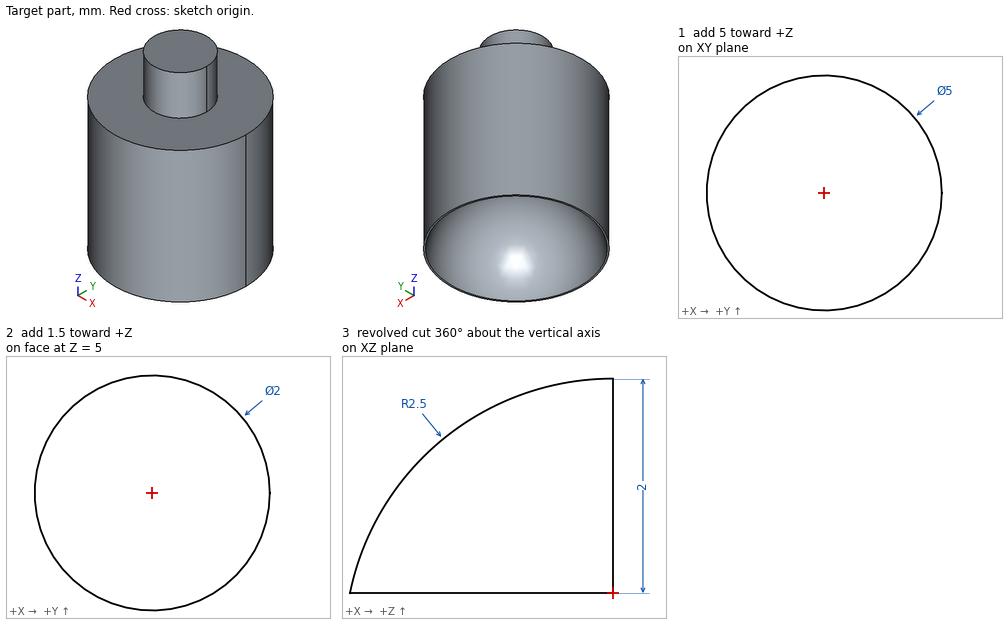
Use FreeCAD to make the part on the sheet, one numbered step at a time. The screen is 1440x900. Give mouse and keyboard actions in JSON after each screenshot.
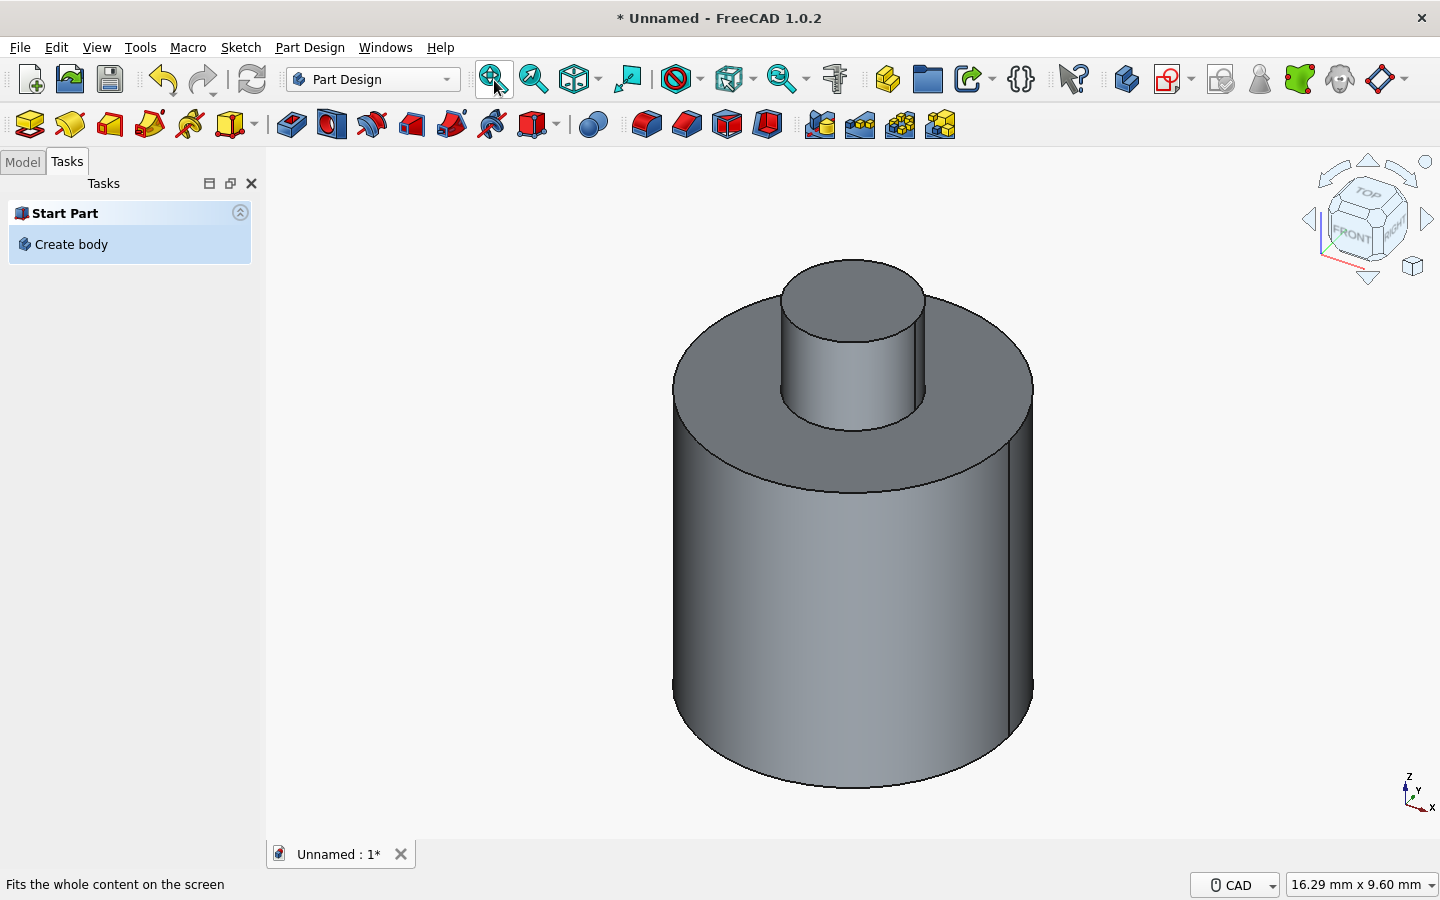
{"action": "left_click", "coordinate": [1168, 80]}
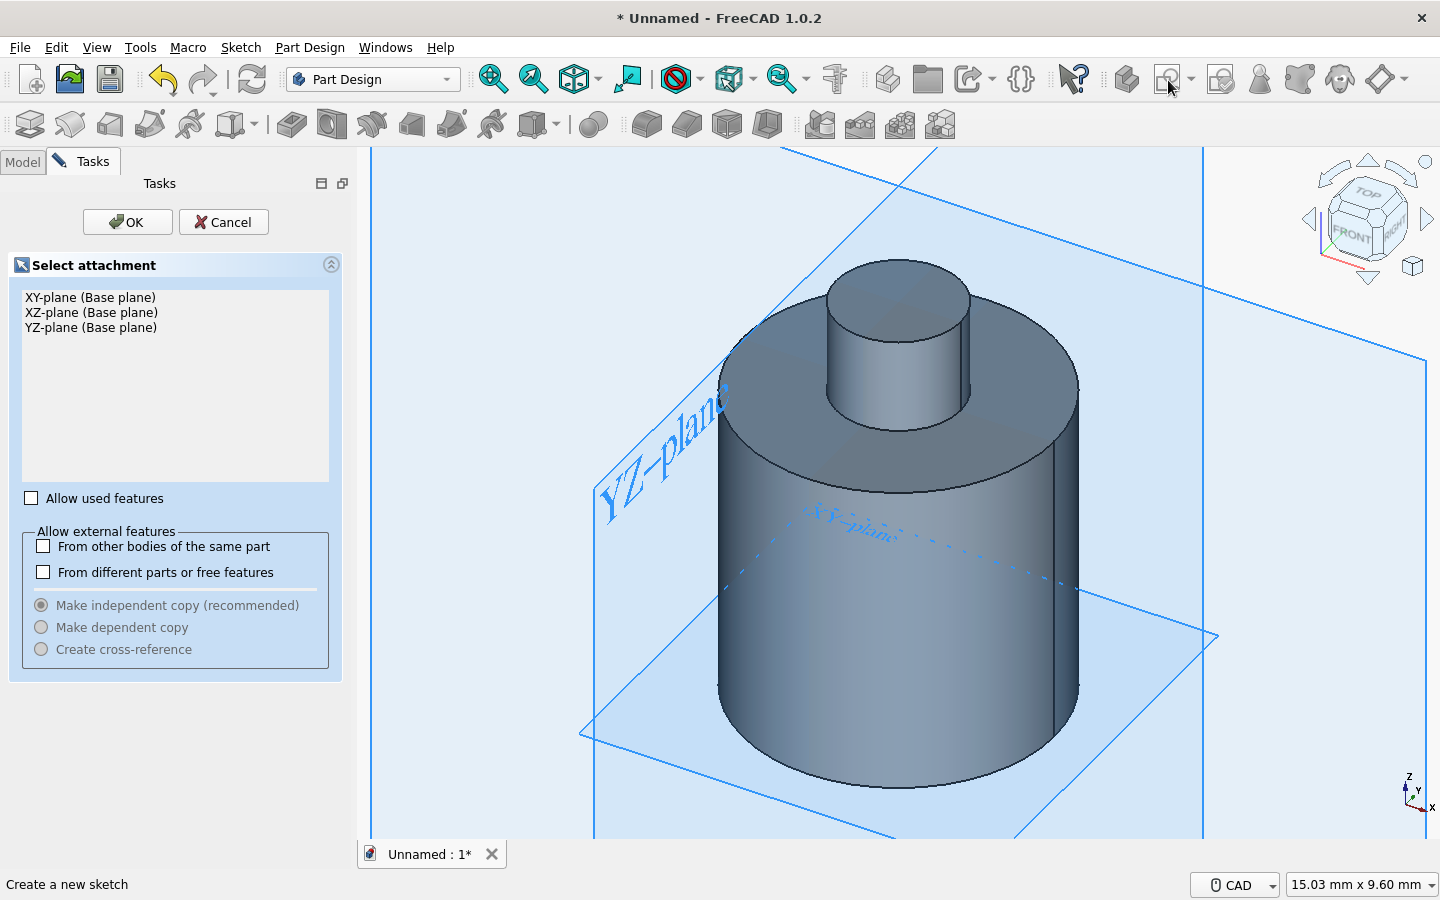
{"action": "left_click", "coordinate": [82, 312]}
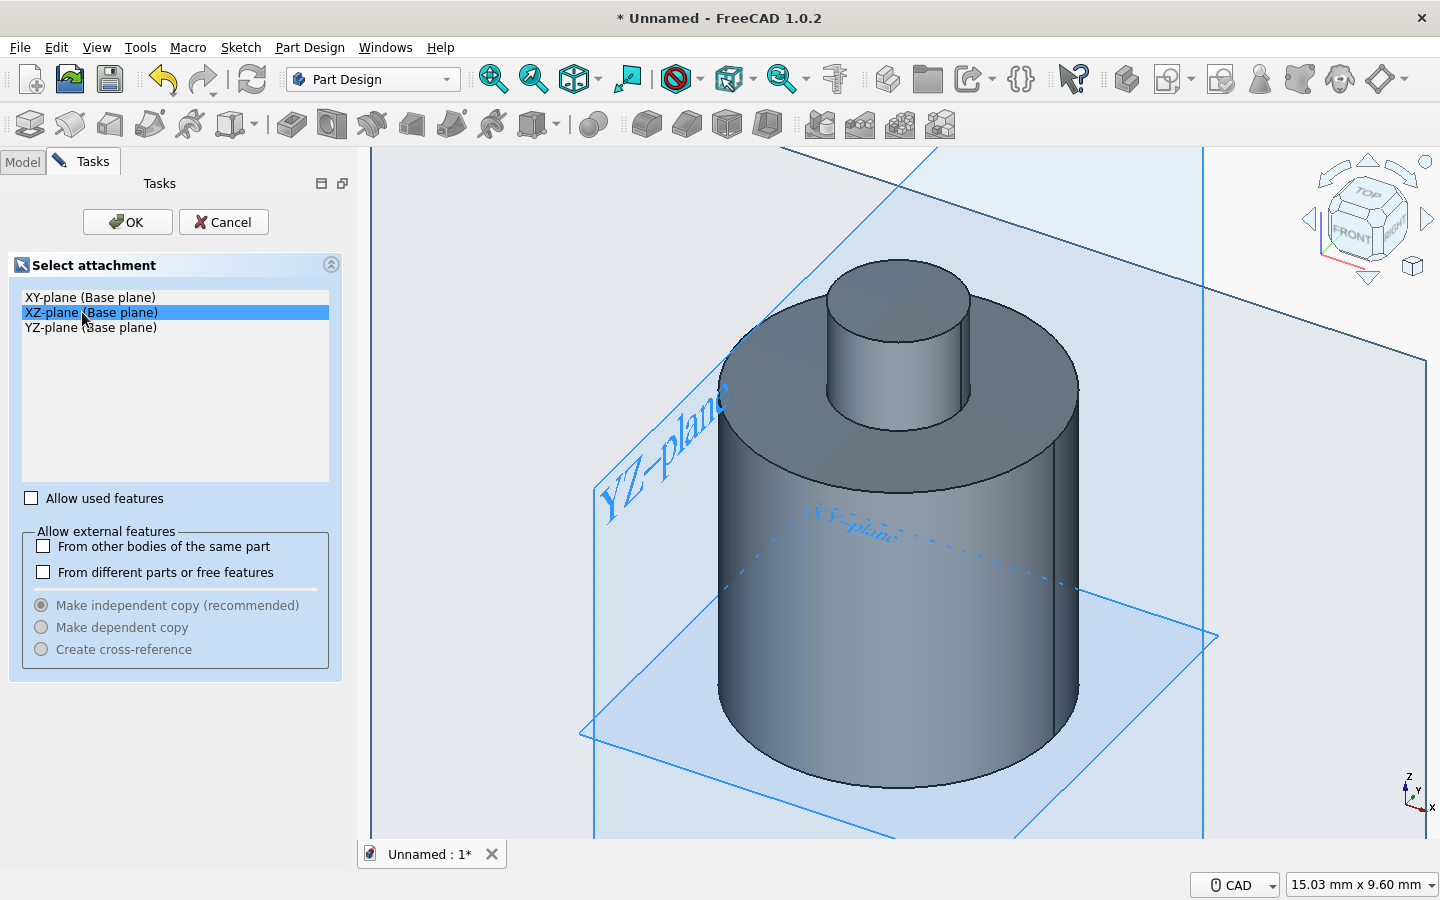
{"action": "left_click", "coordinate": [128, 222]}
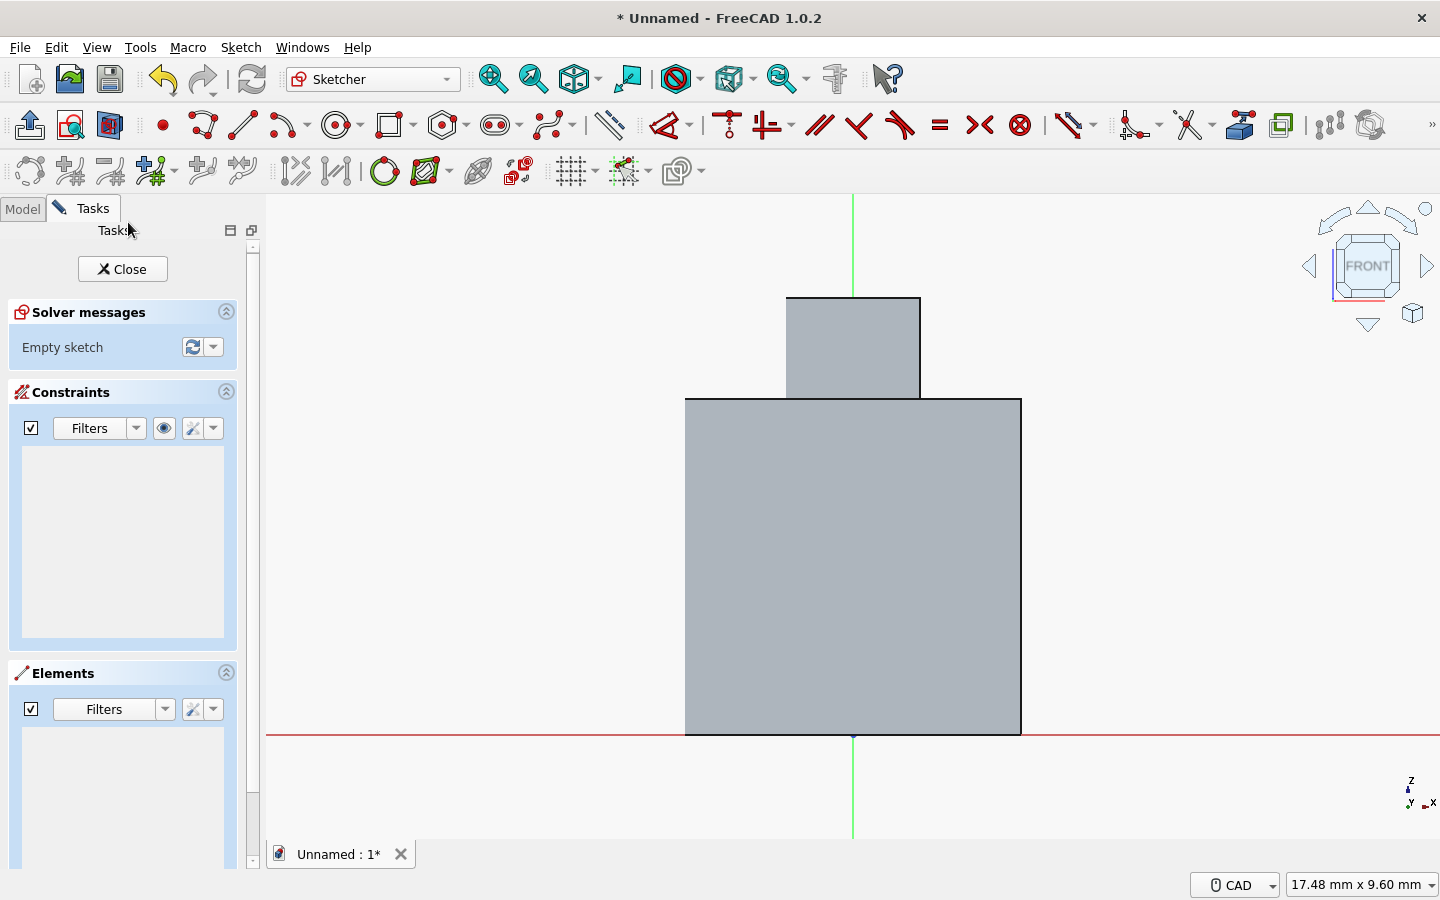
{"action": "left_click", "coordinate": [110, 126]}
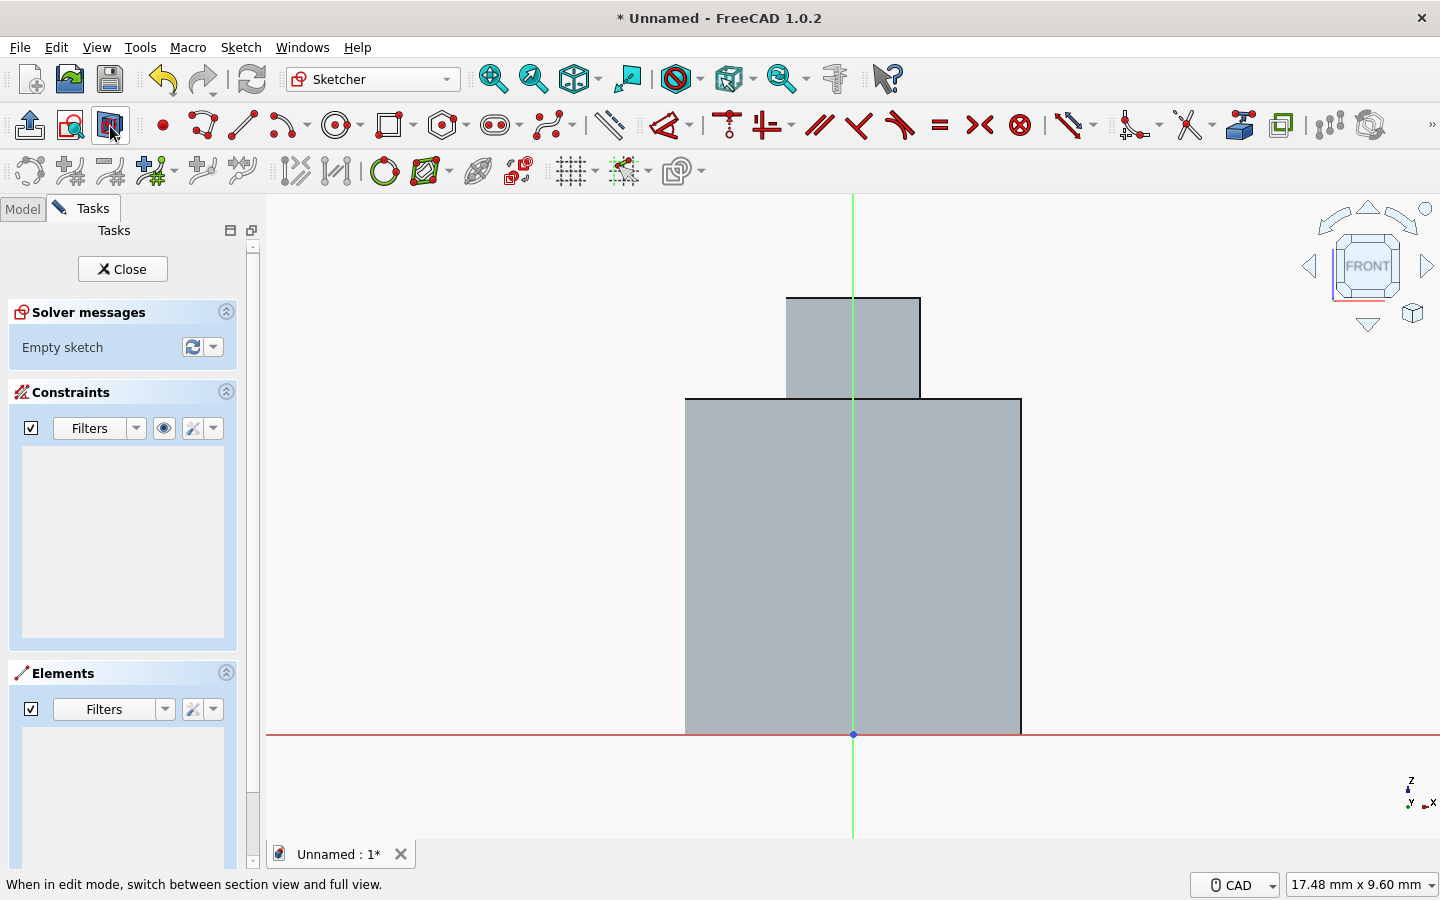
{"action": "scroll", "coordinate": [765, 733], "scroll_direction": "up", "scroll_amount": 6}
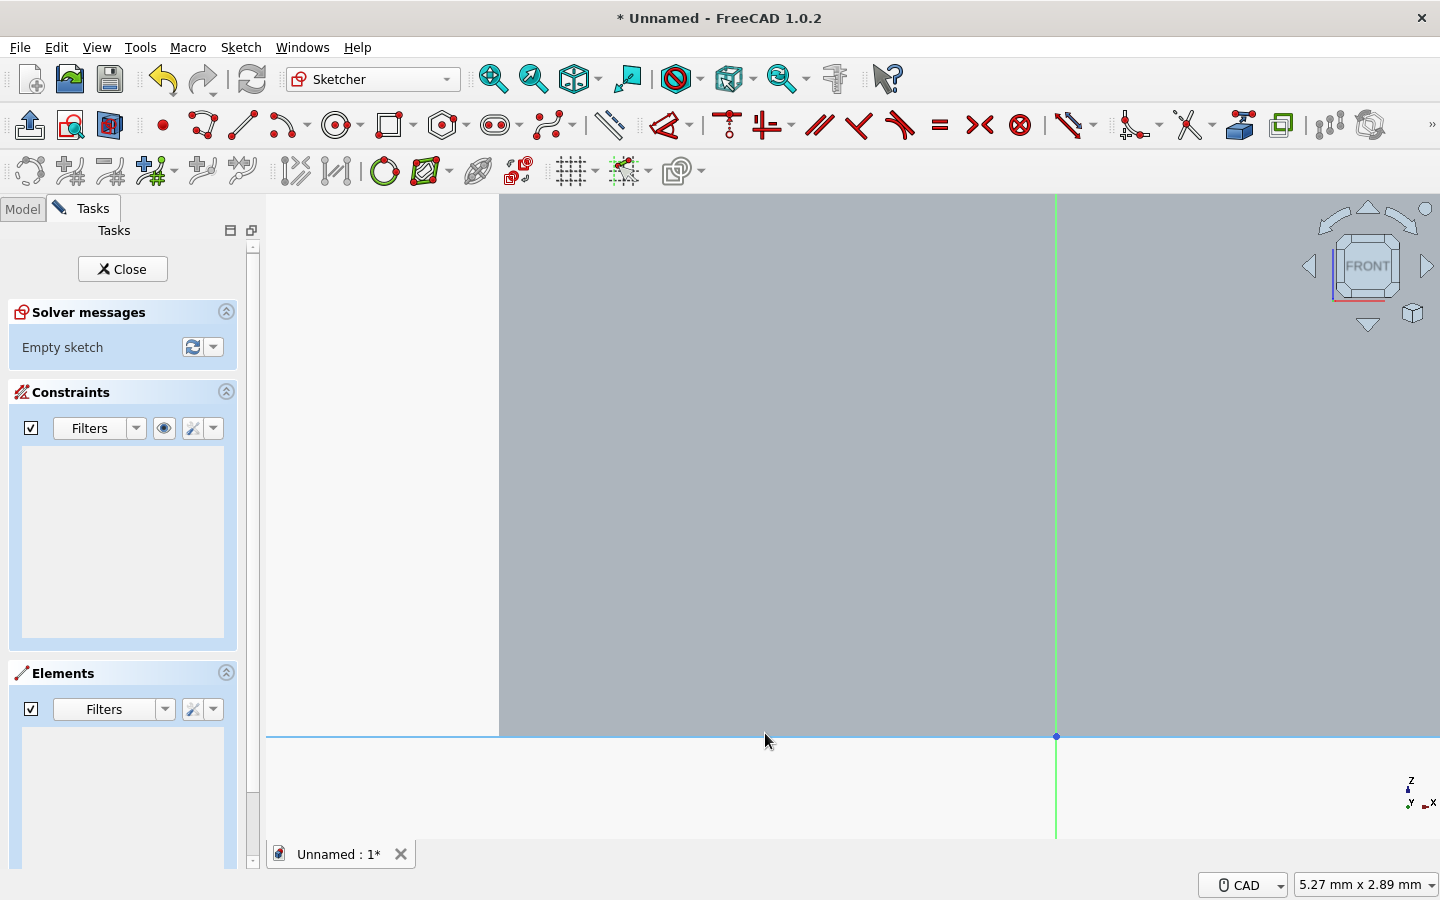
{"action": "left_click", "coordinate": [204, 126]}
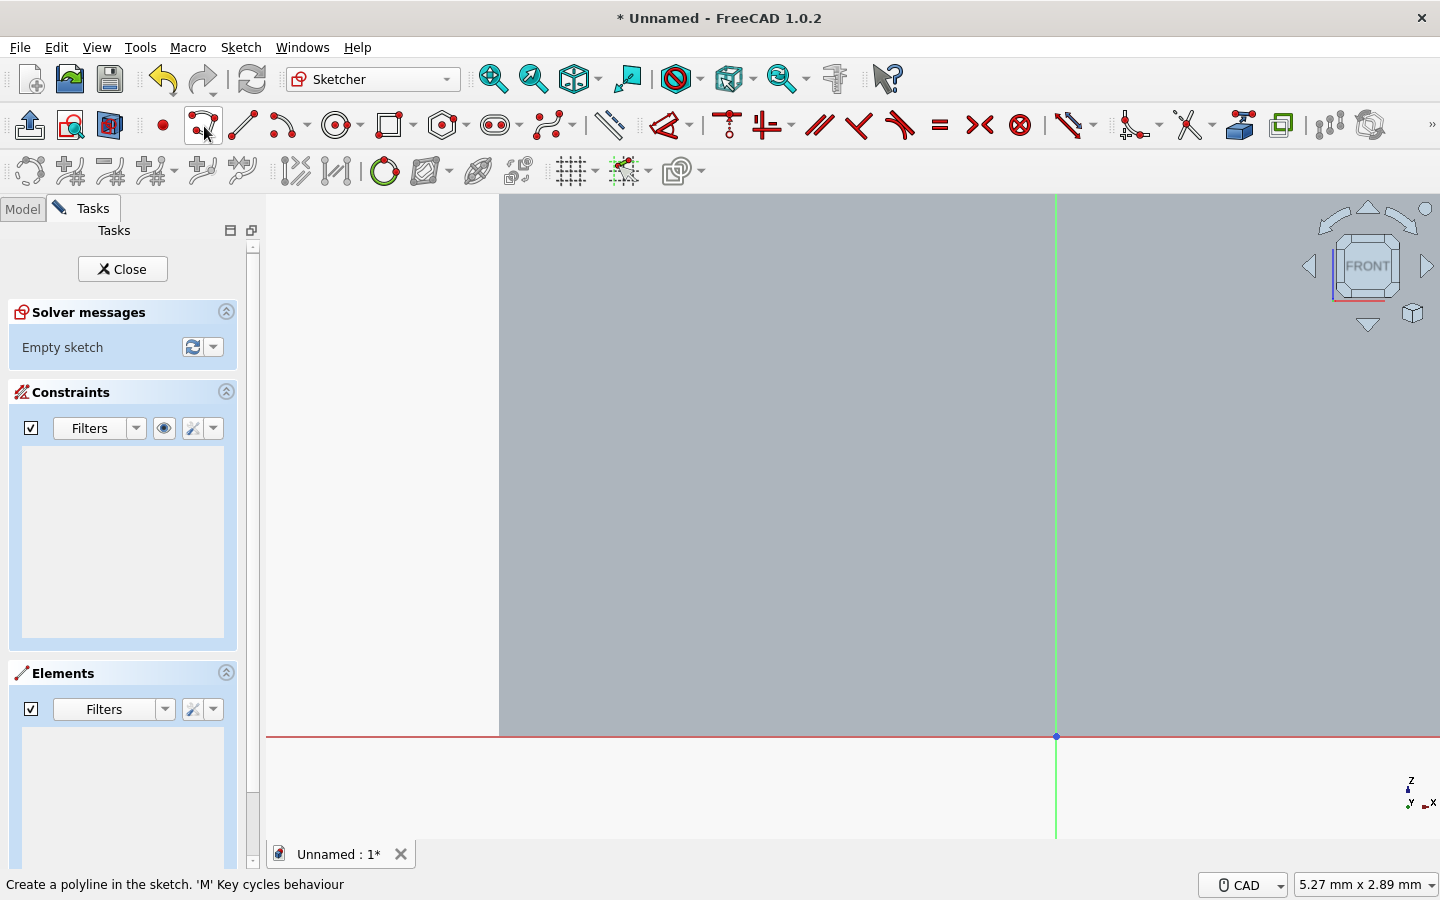
{"action": "left_click", "coordinate": [1056, 291]}
{"action": "left_click", "coordinate": [1056, 737]}
{"action": "left_click", "coordinate": [510, 728]}
{"action": "right_click", "coordinate": [510, 728]}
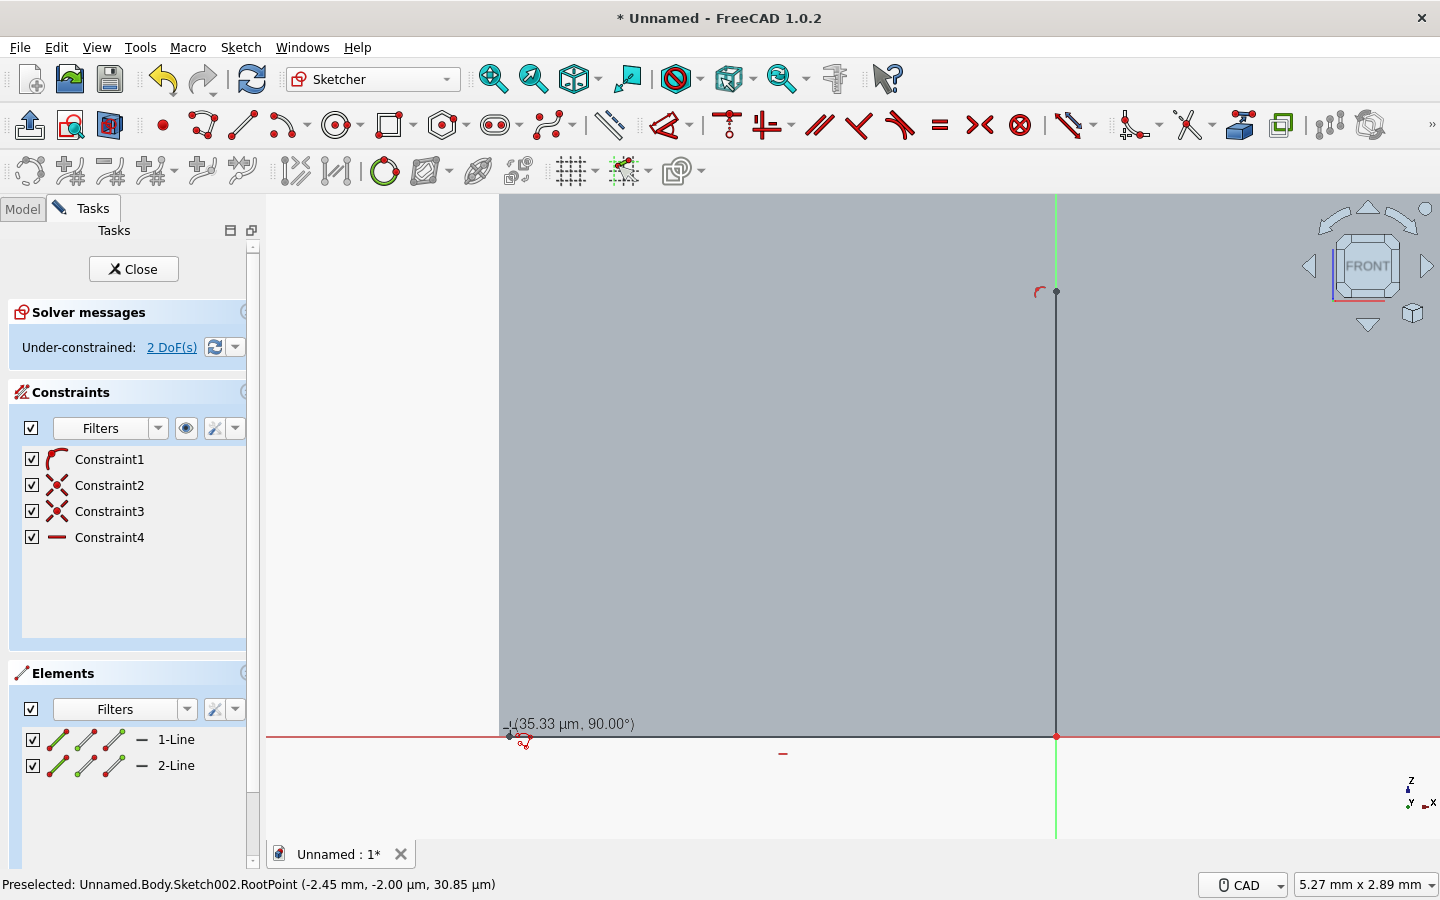
{"action": "key", "text": "g 3 a"}